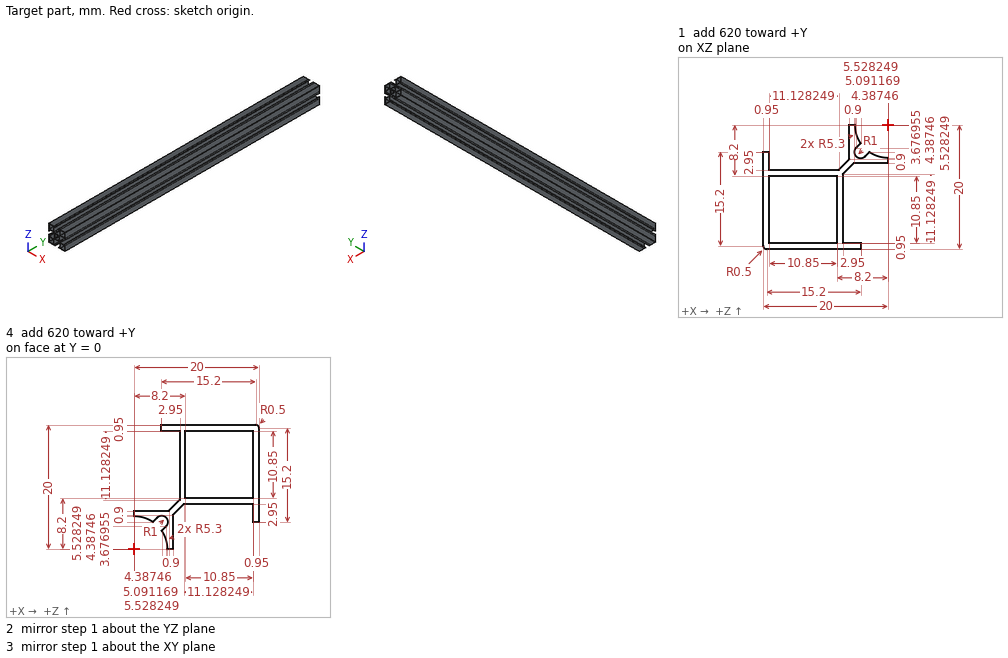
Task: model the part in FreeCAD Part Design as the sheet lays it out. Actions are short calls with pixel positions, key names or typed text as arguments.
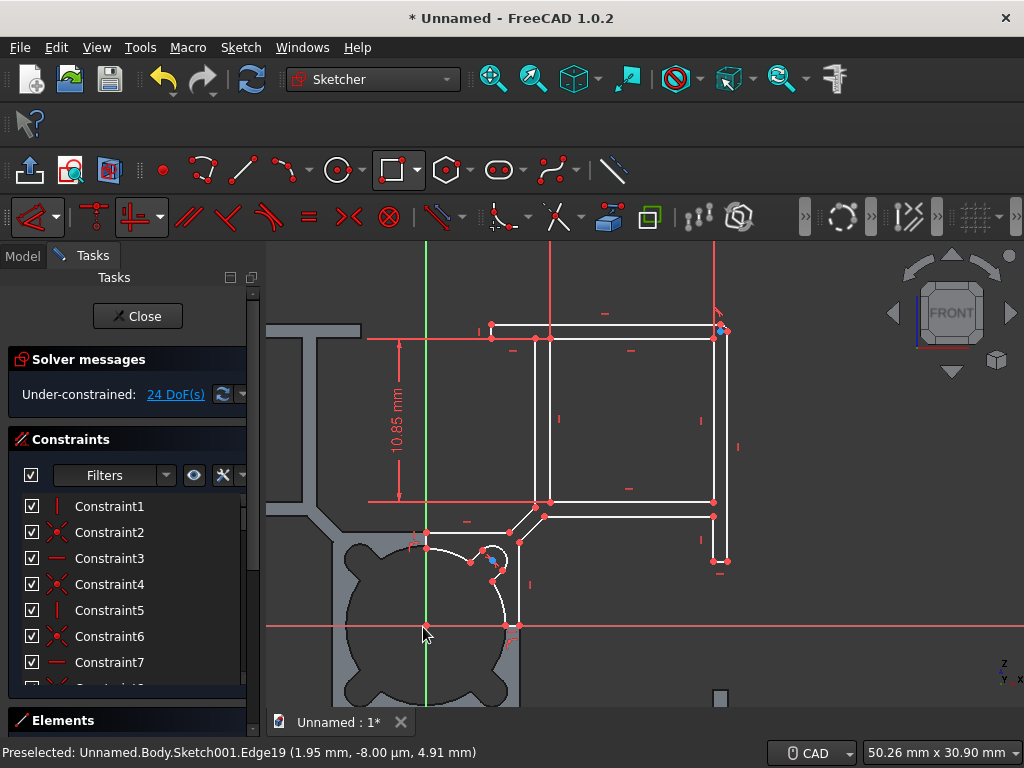
click(504, 612)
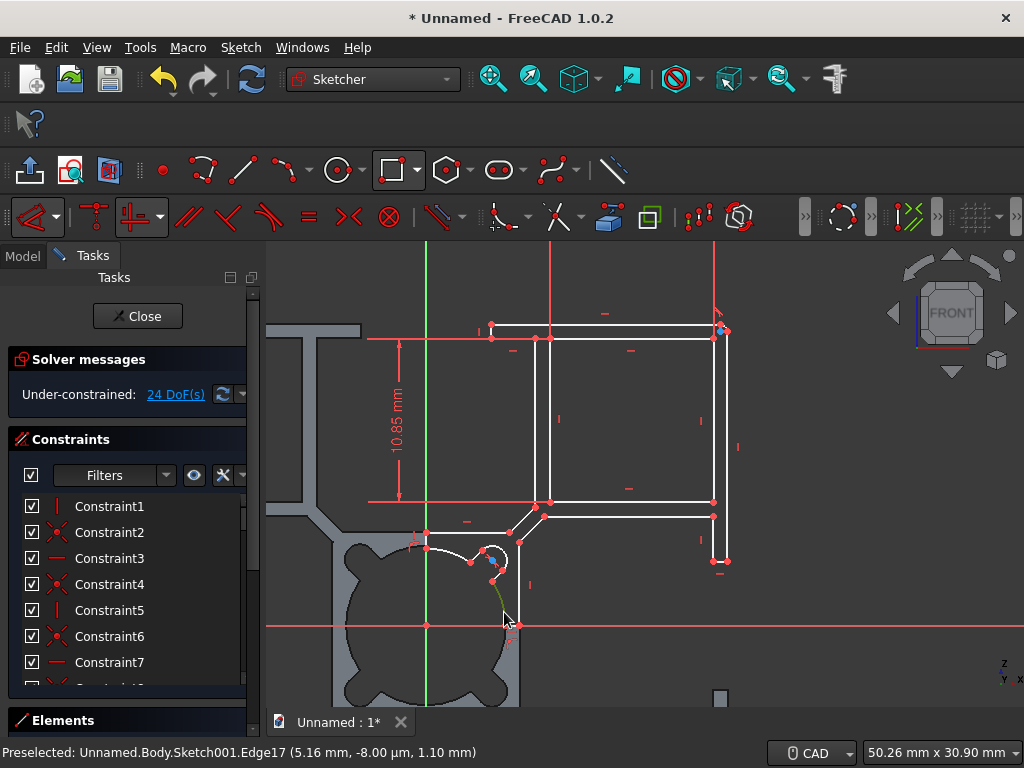
click(458, 556)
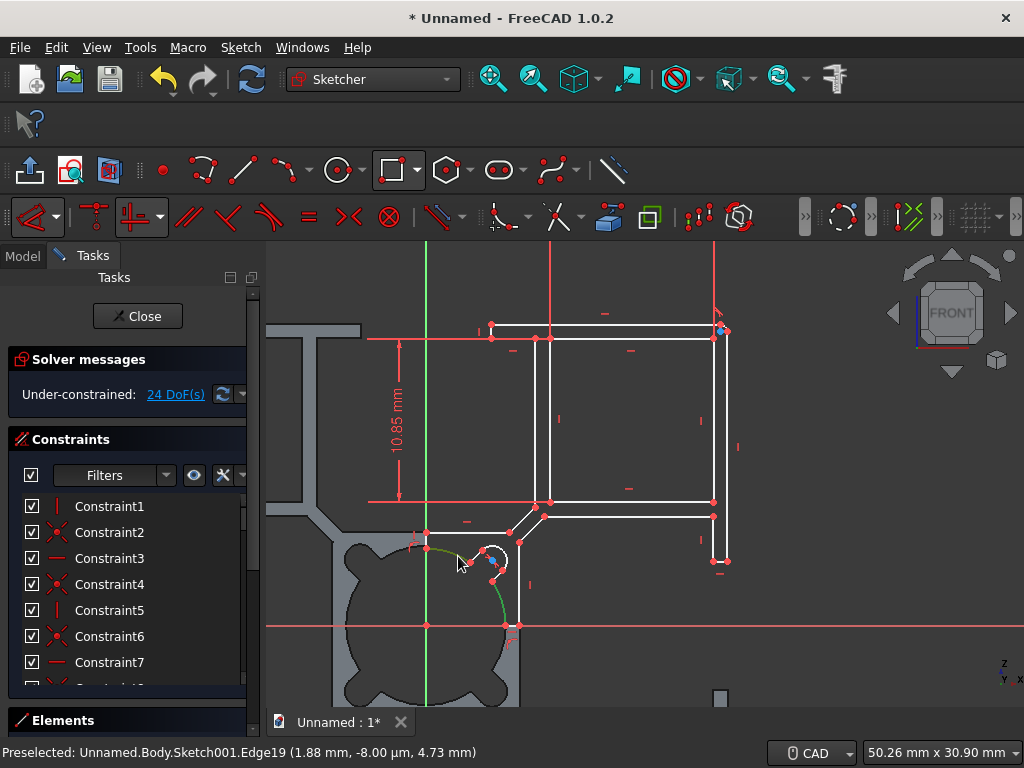
click(310, 218)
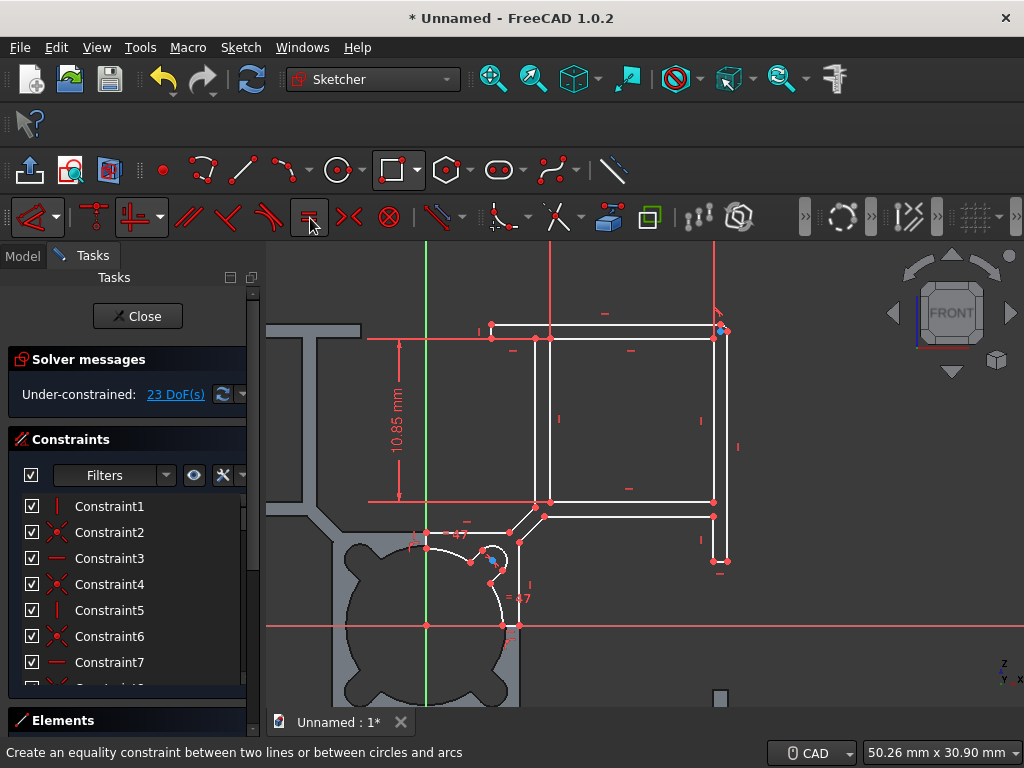
click(502, 612)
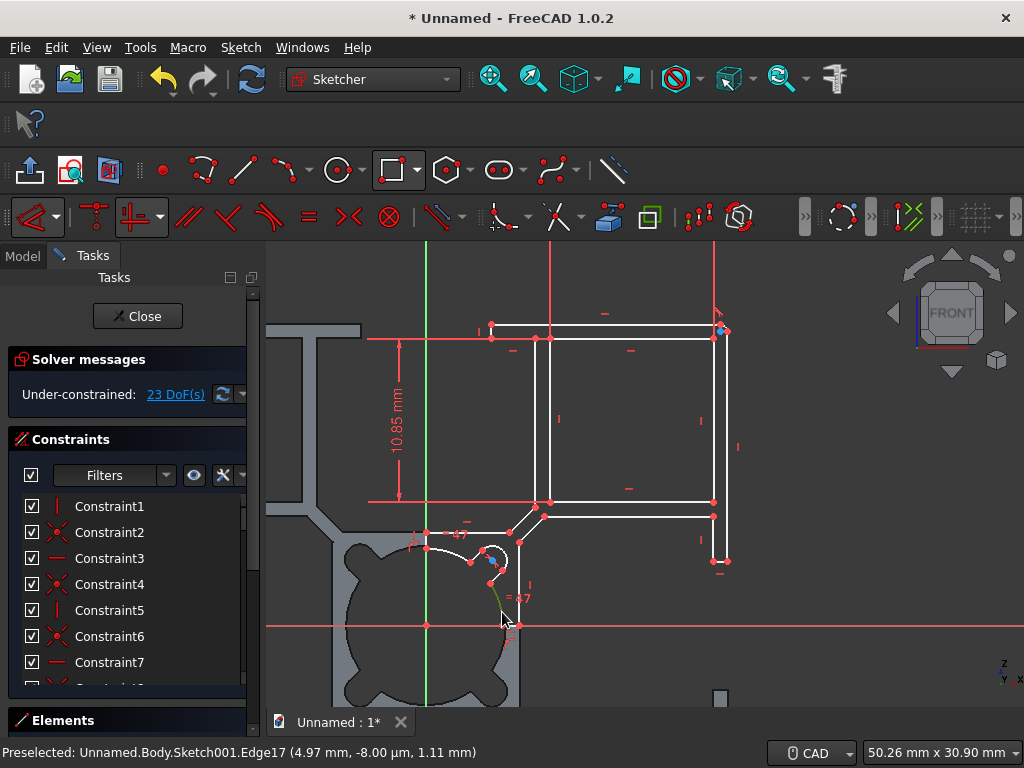
click(58, 218)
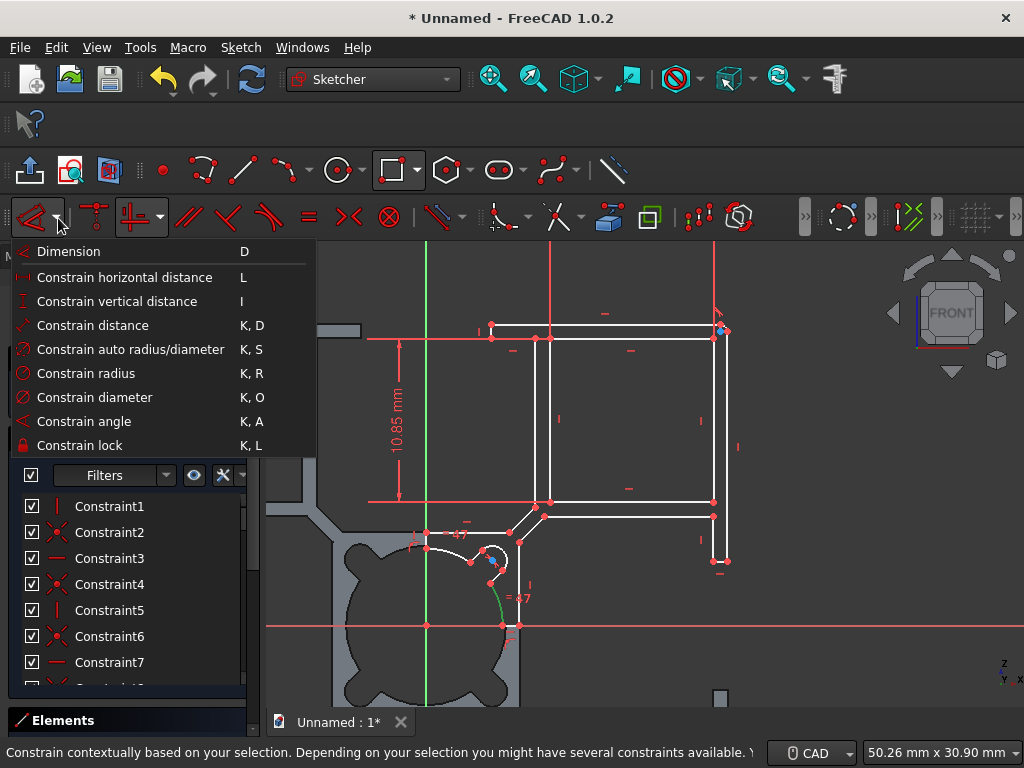
click(164, 373)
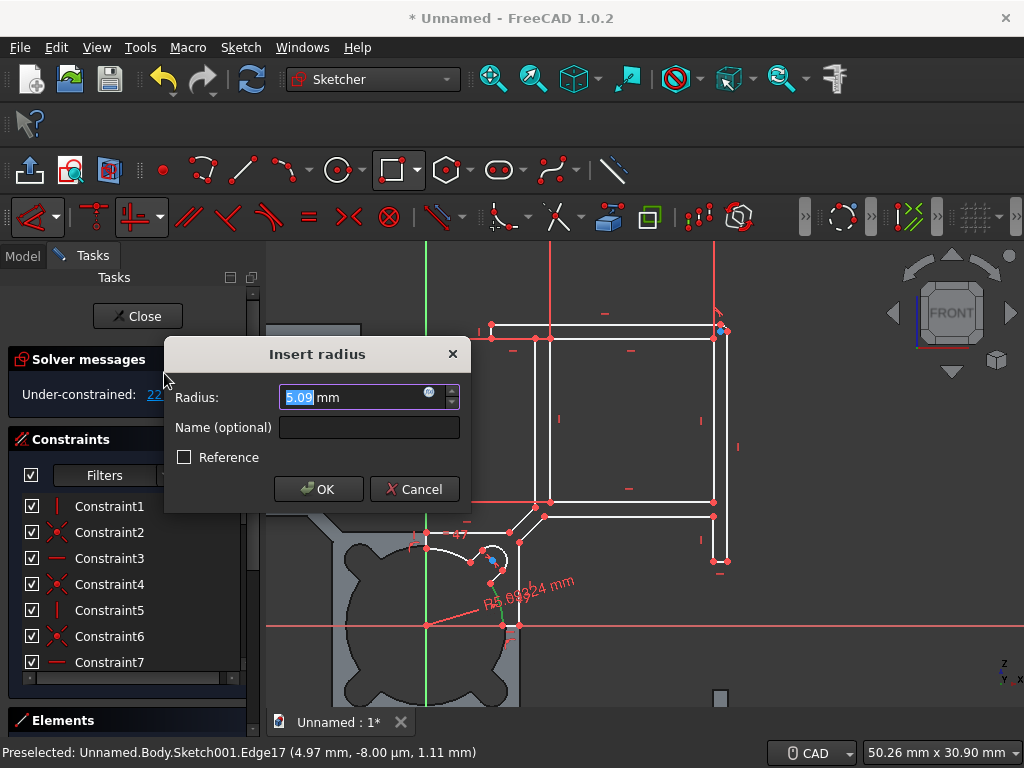
text(5.3)
key(Return)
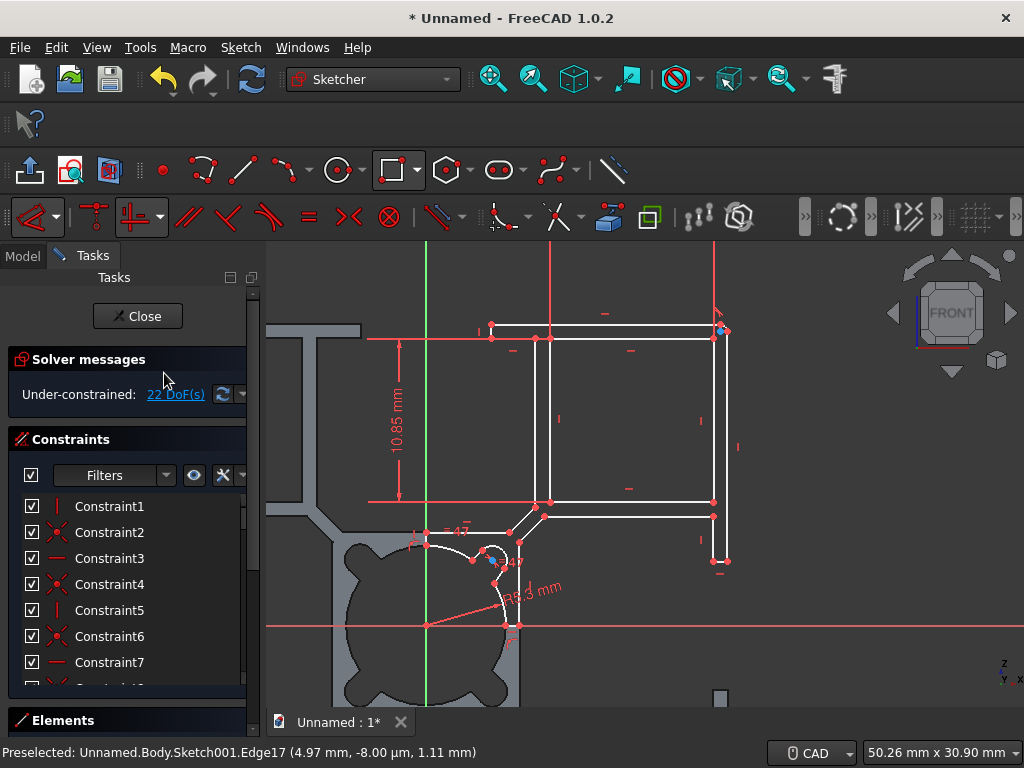
scroll(506, 557, up, 5)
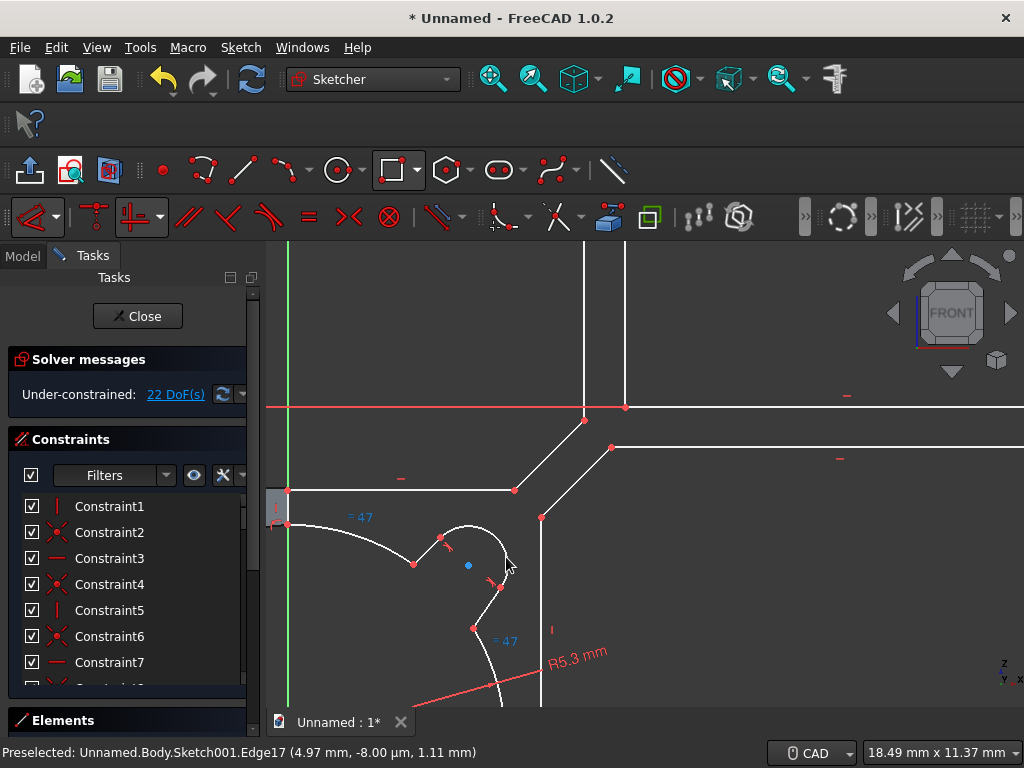
click(506, 555)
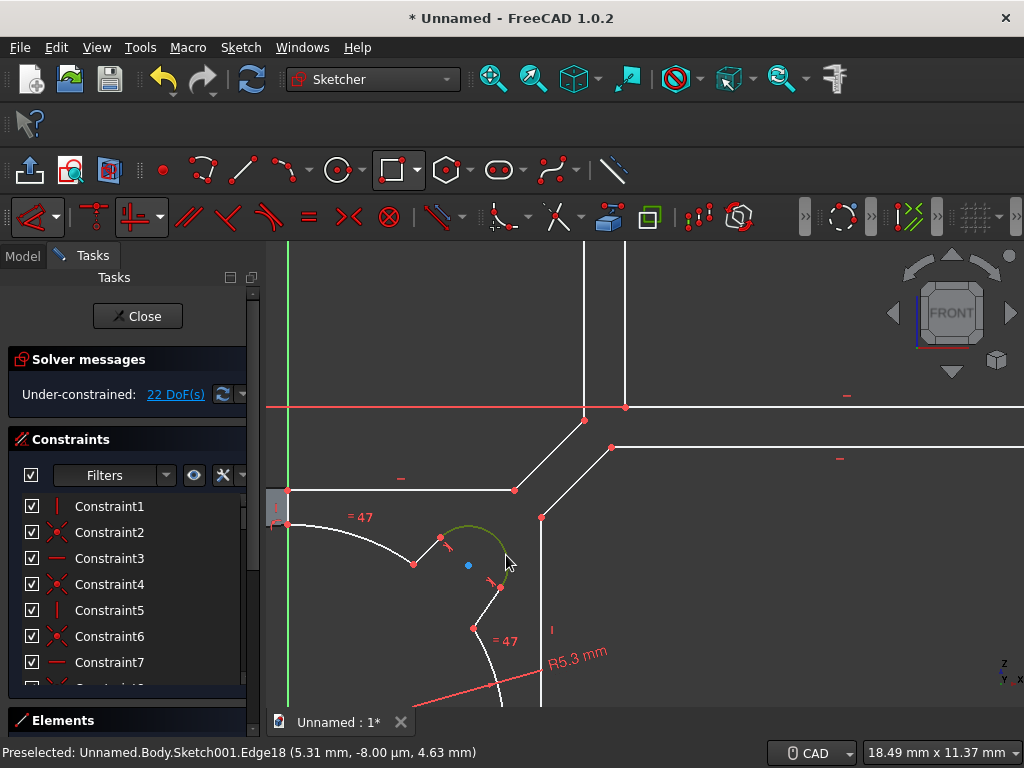
click(58, 218)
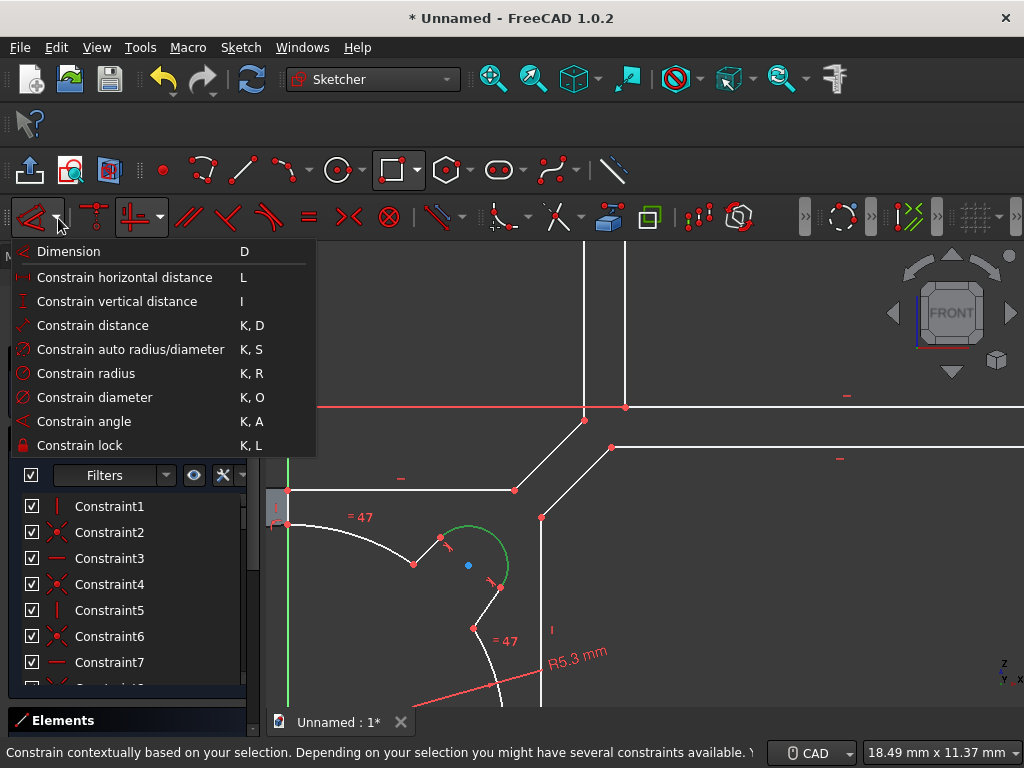
click(164, 373)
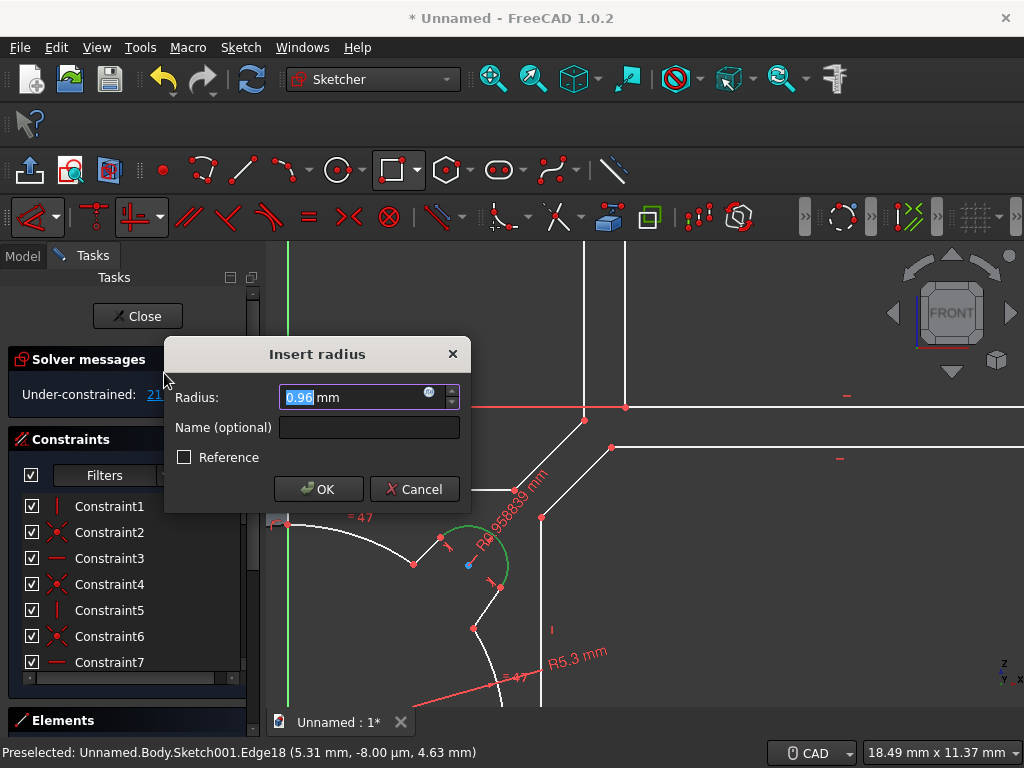
text(1)
key(Return)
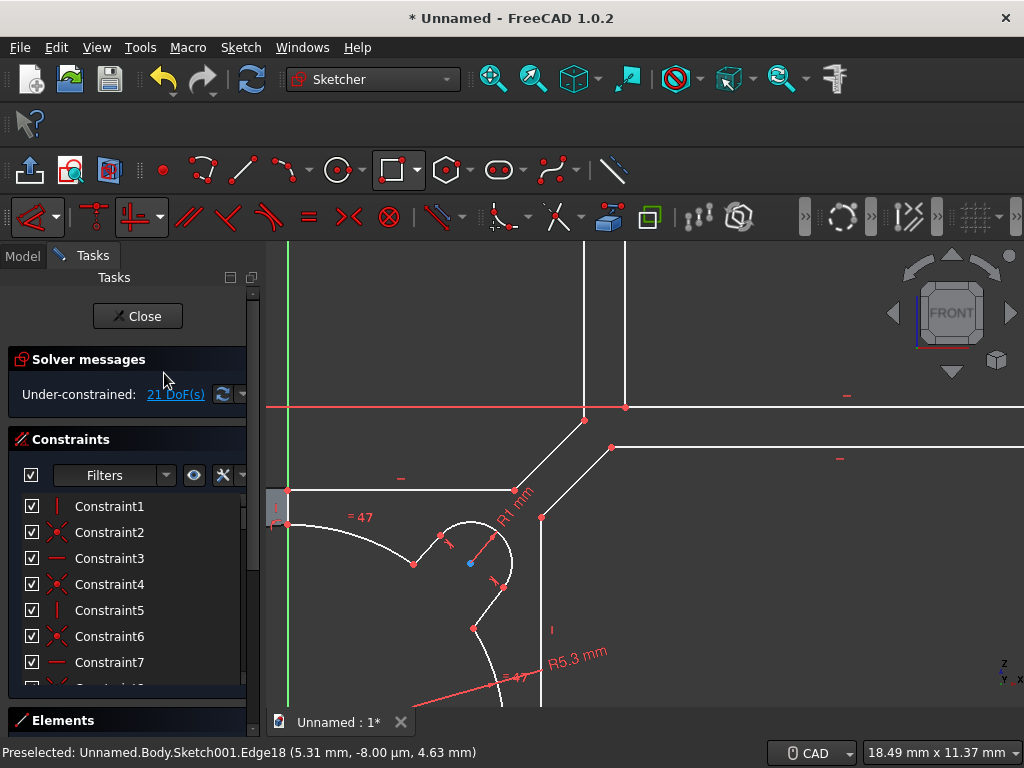
scroll(506, 557, down, 5)